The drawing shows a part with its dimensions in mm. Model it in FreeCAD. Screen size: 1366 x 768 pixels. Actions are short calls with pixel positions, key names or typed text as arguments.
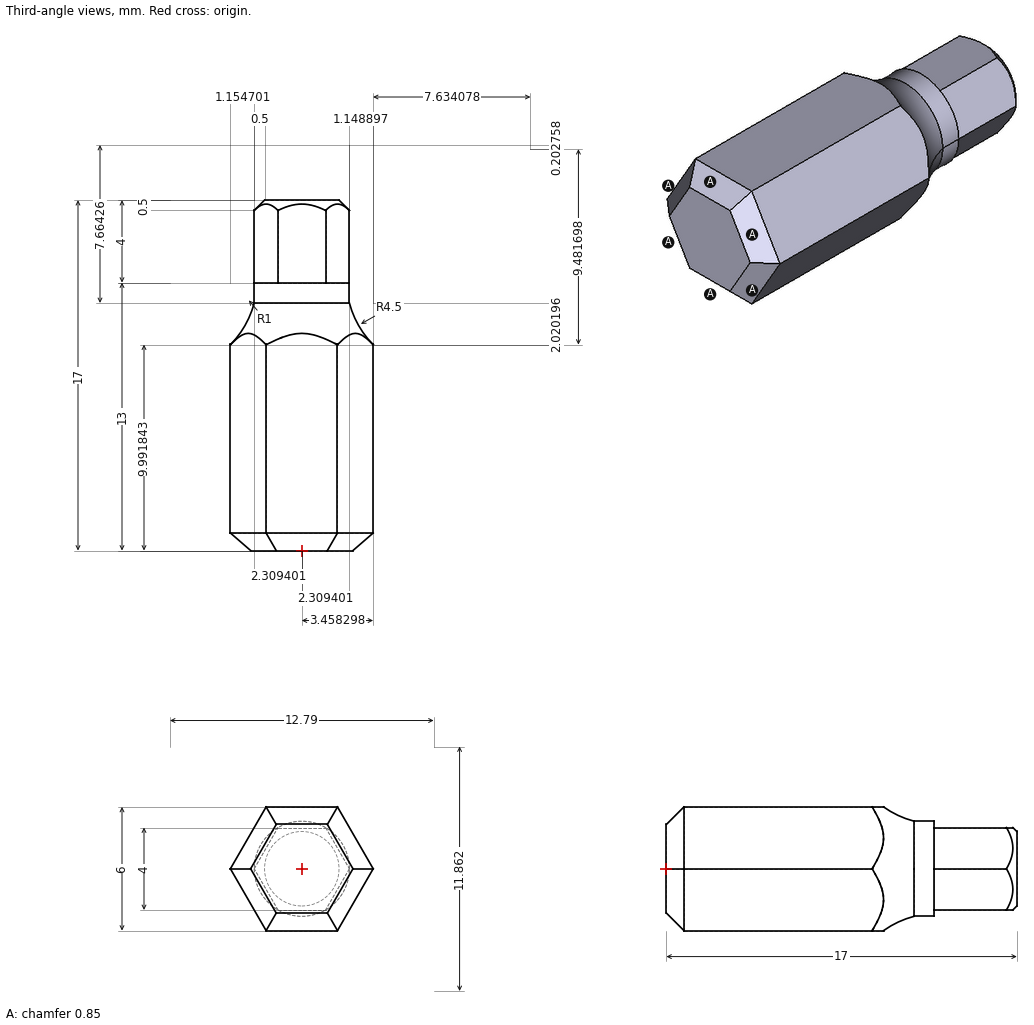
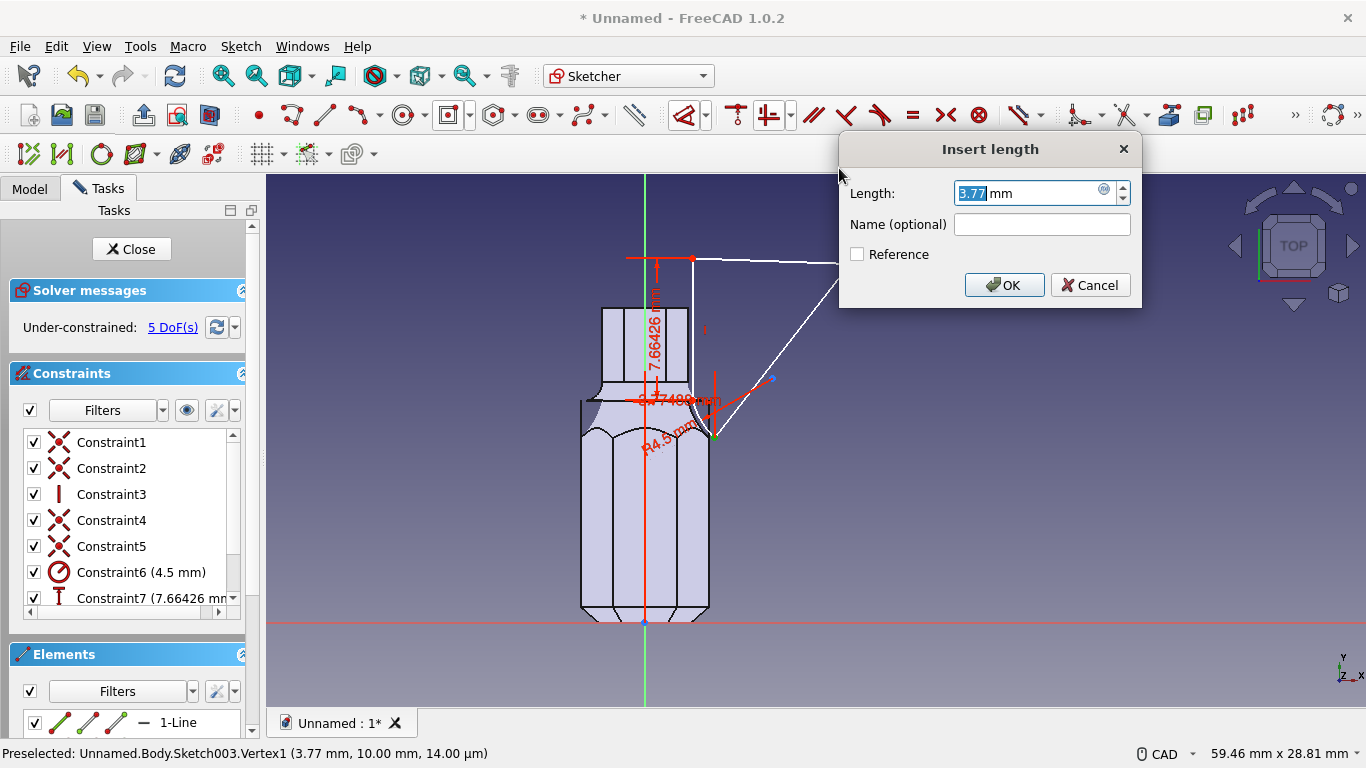
text(3.458298)
key(Return)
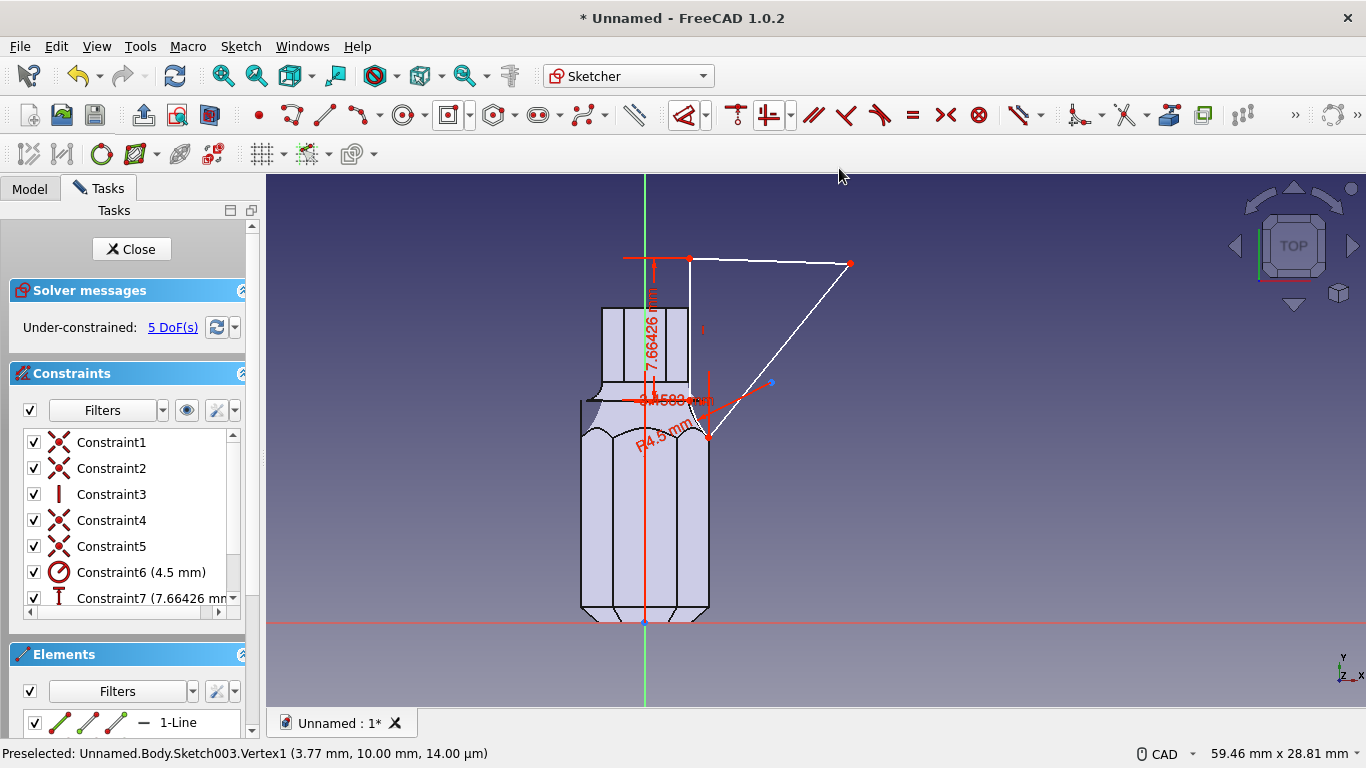
click(709, 438)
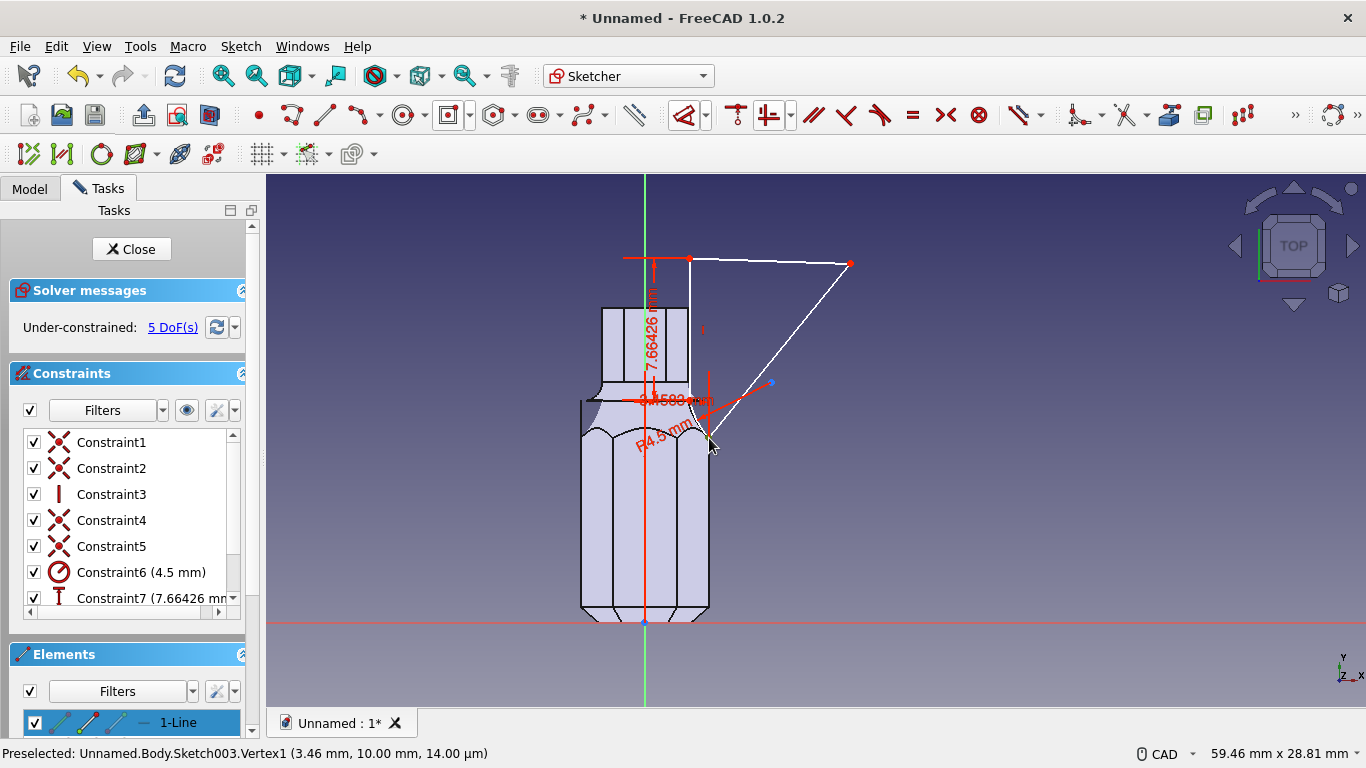
key(i)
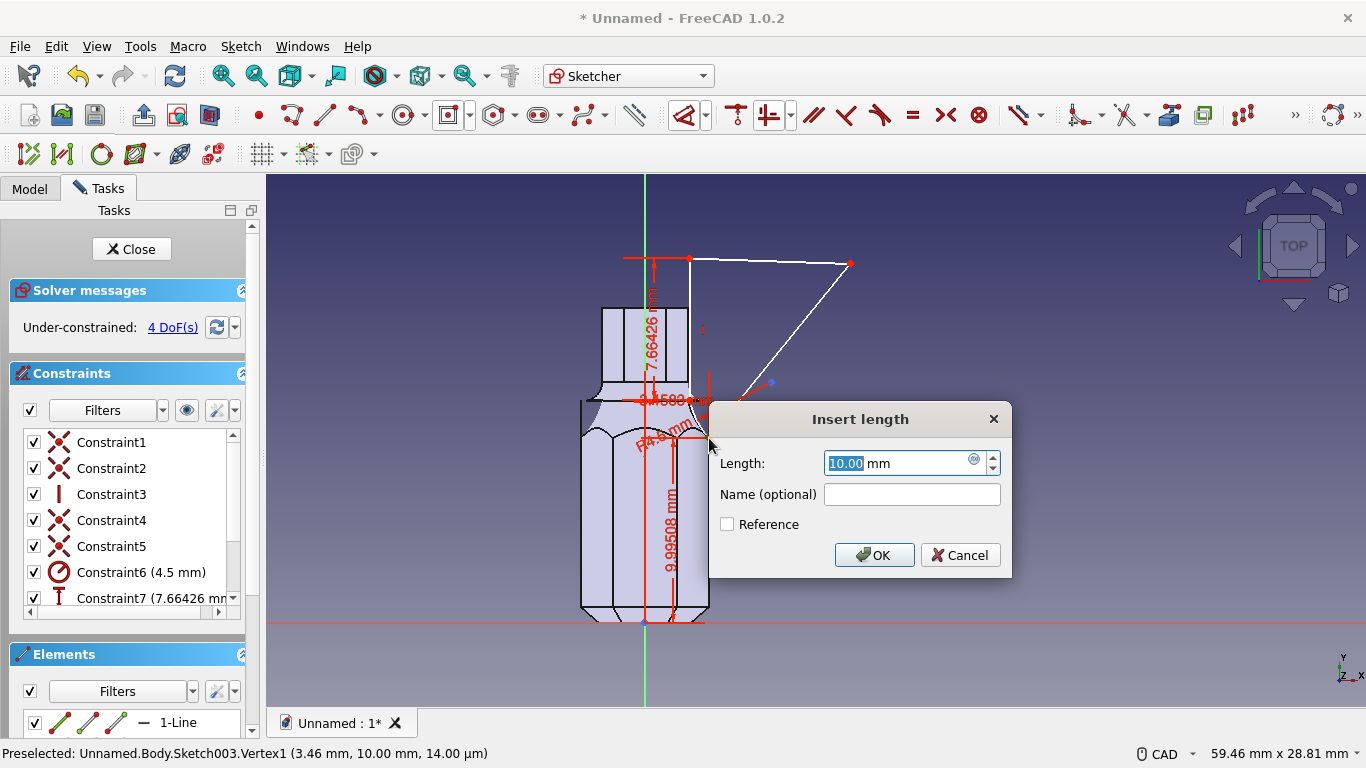
text(9.991843)
key(Return)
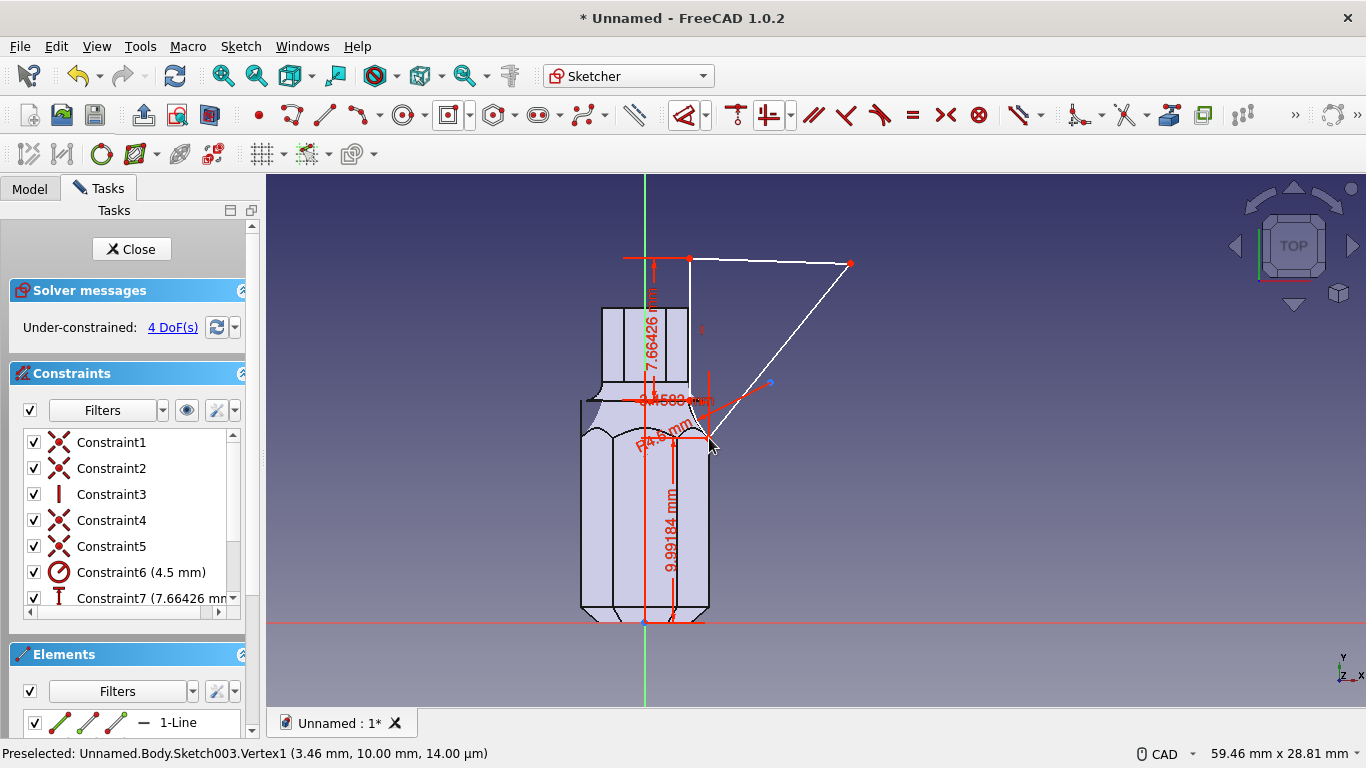
click(690, 258)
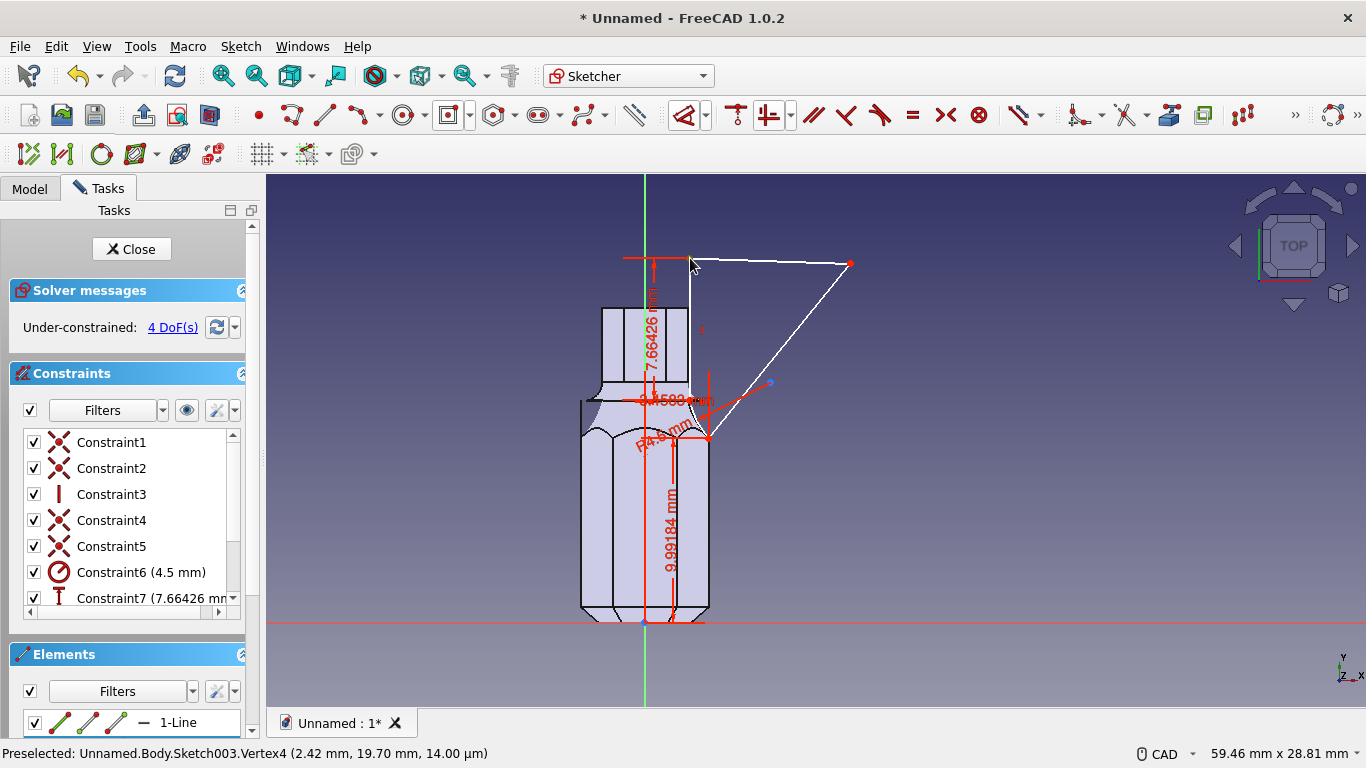
key(l)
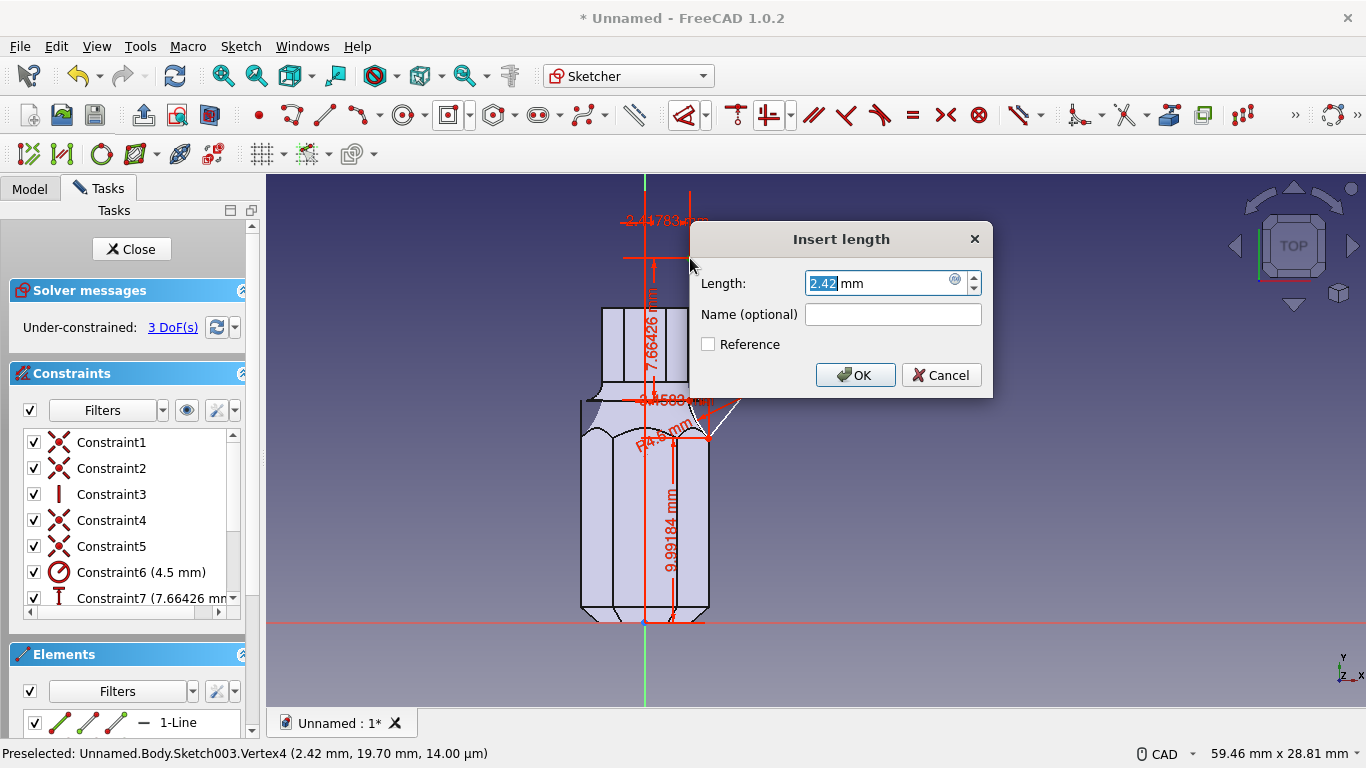
text(2.309401)
key(Return)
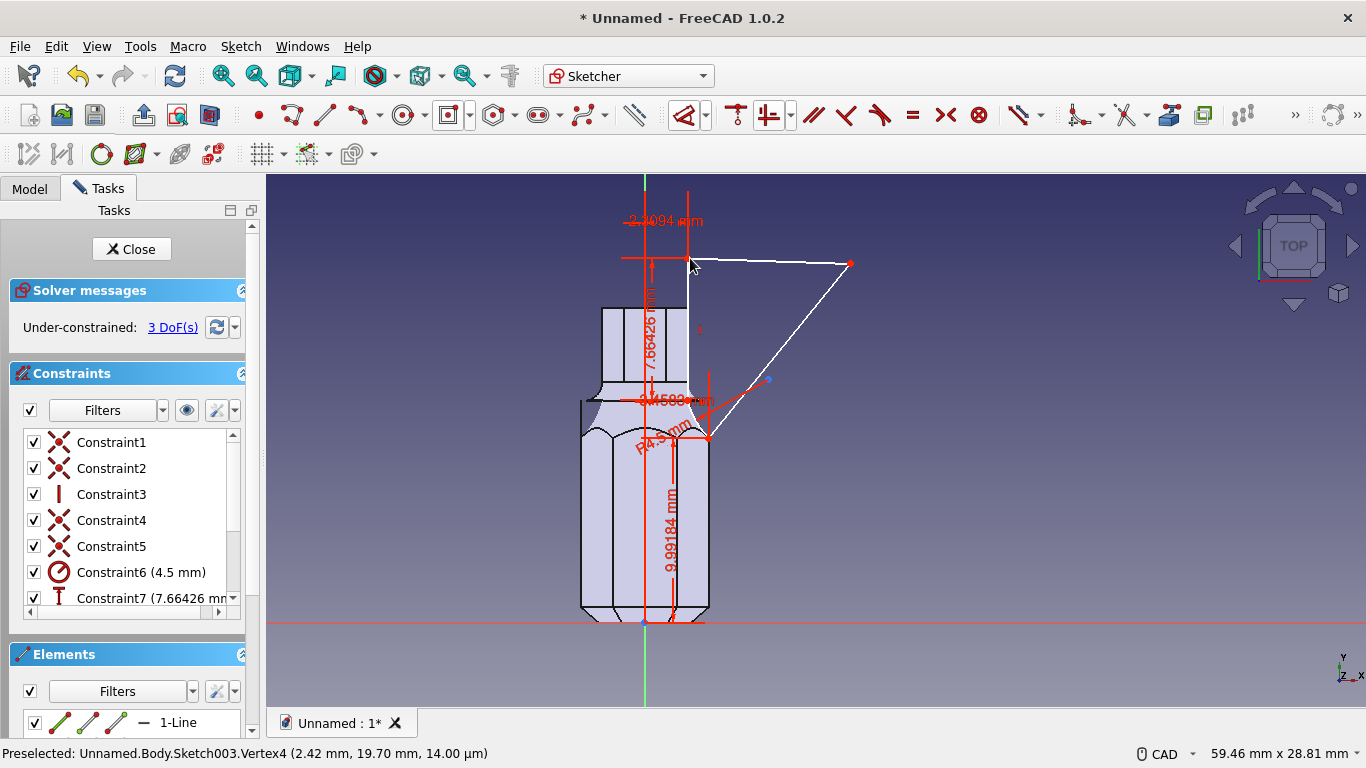
click(751, 386)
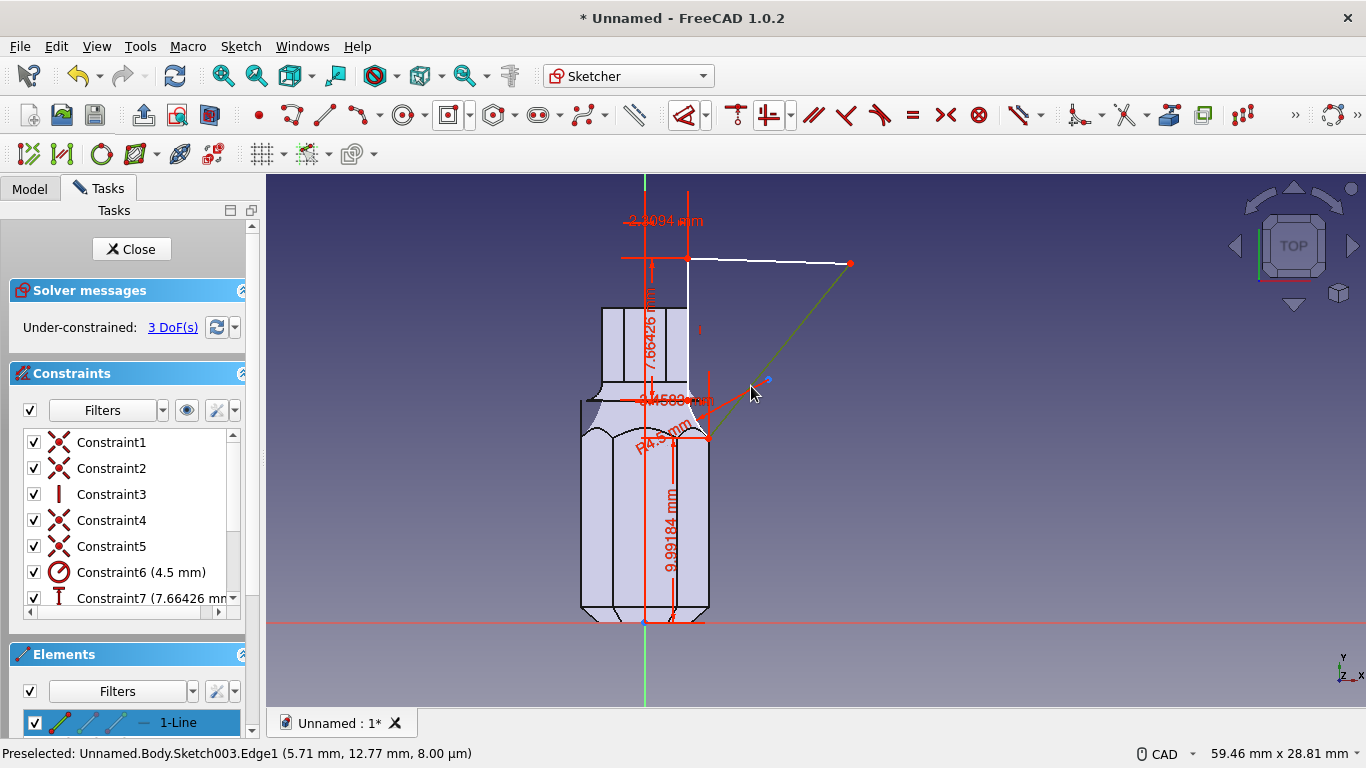
key(l)